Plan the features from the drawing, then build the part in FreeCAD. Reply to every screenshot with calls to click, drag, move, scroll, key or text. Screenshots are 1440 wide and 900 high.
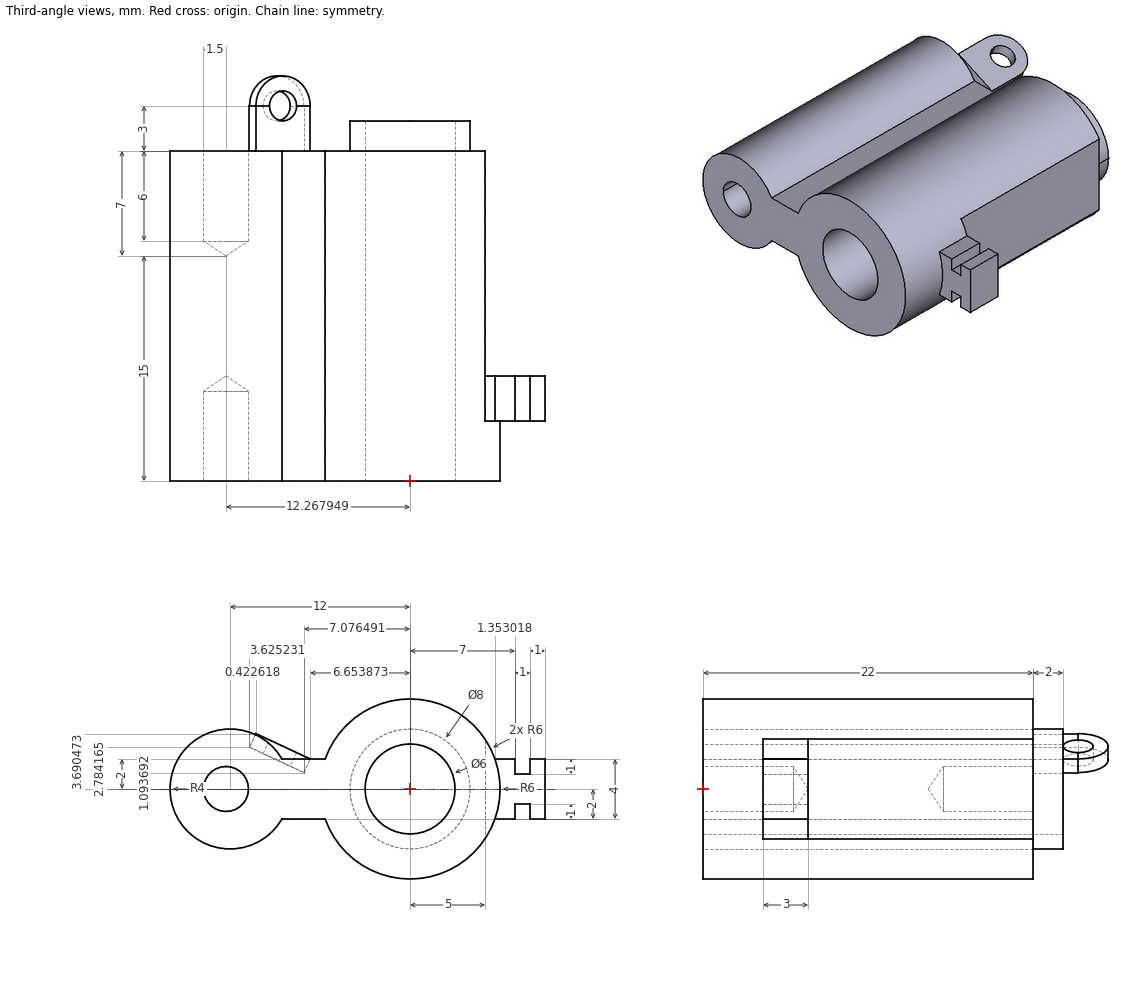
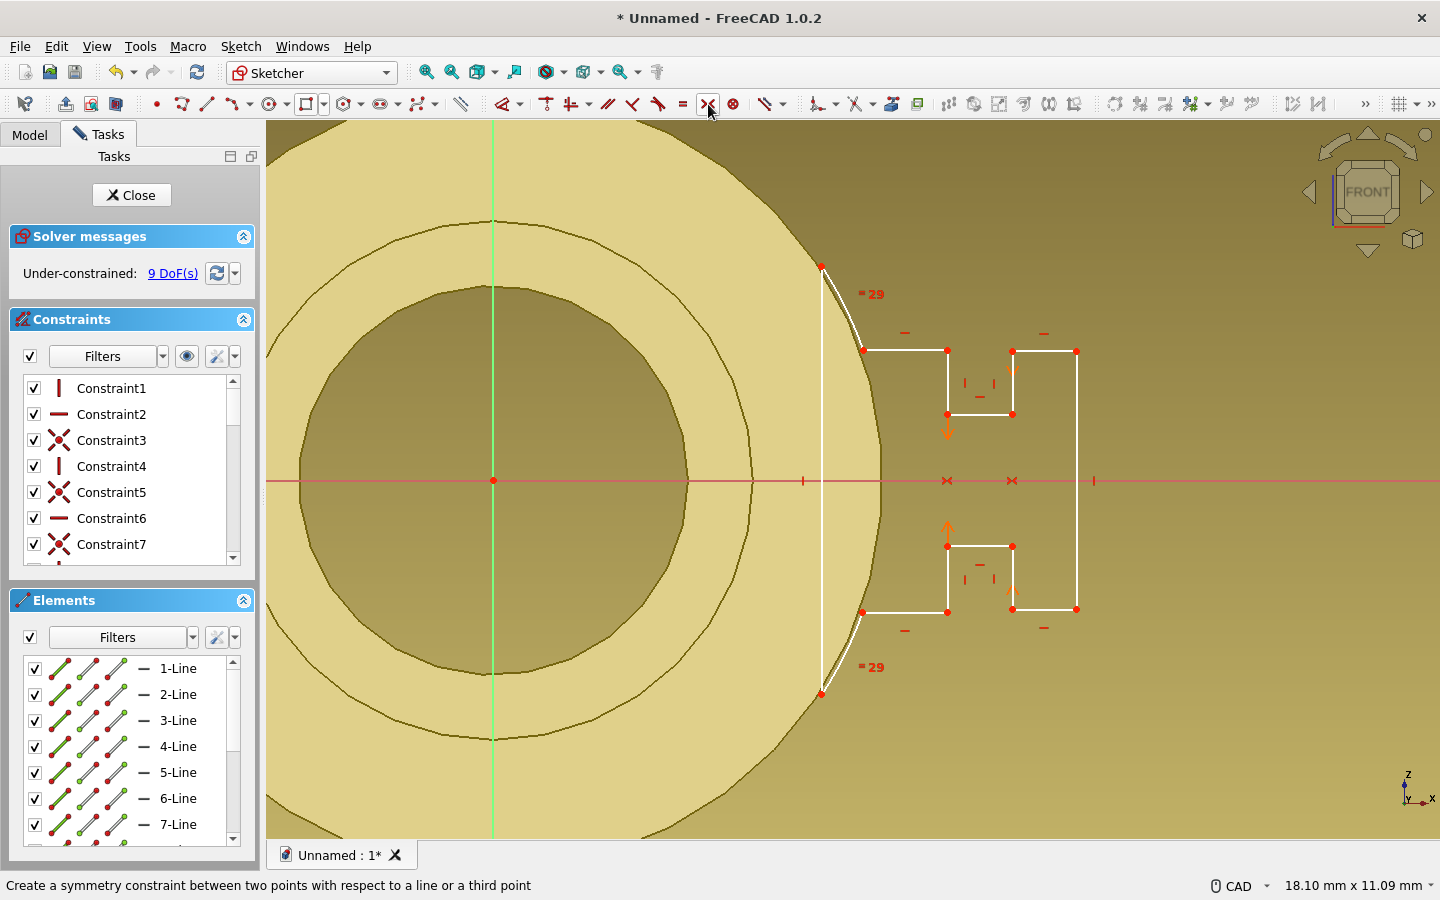
click(502, 104)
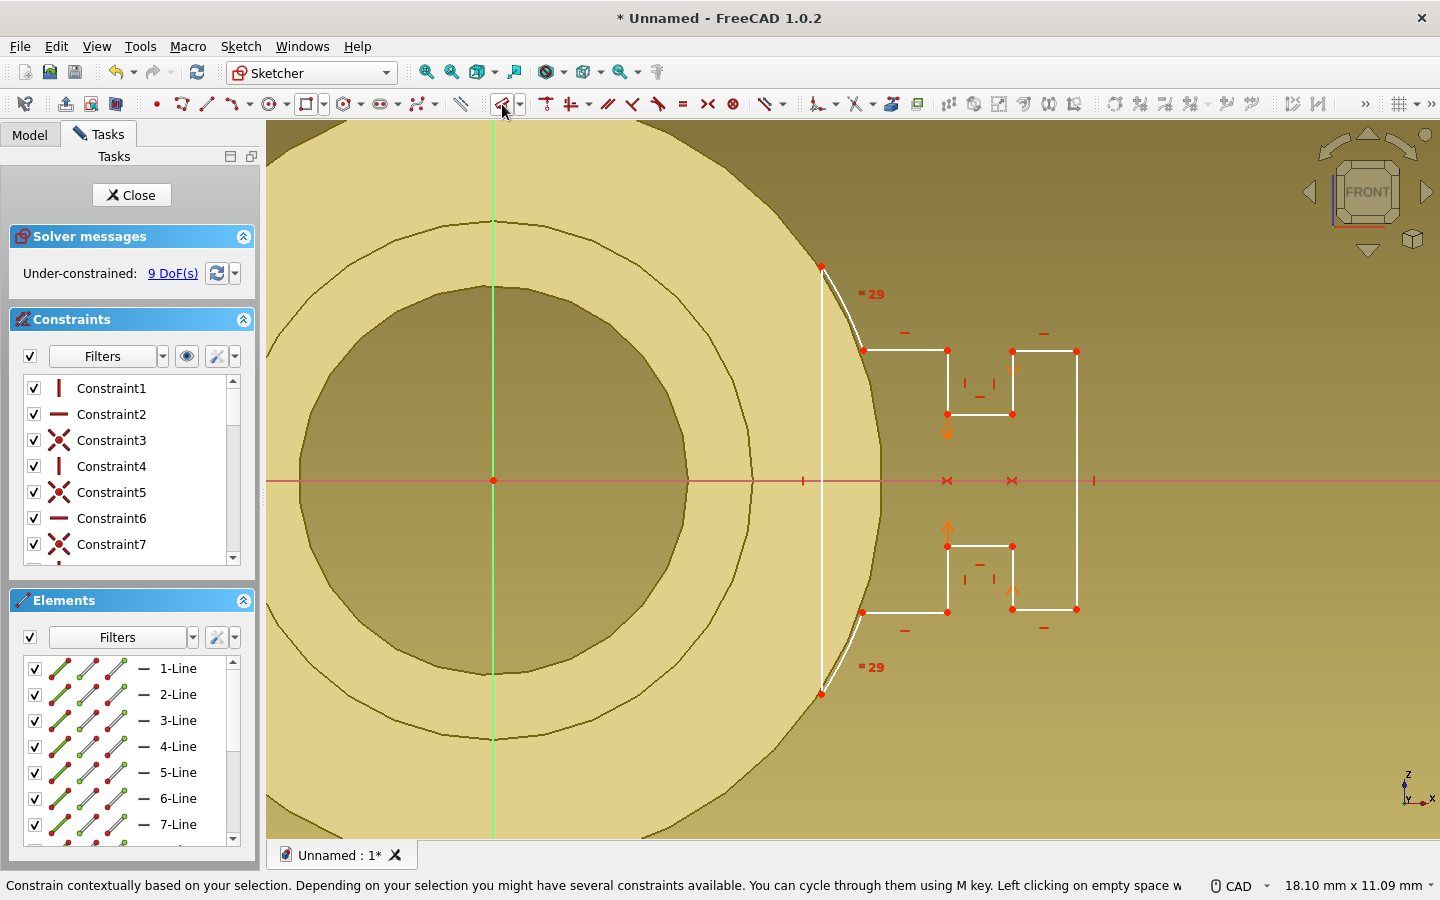
click(853, 324)
click(882, 311)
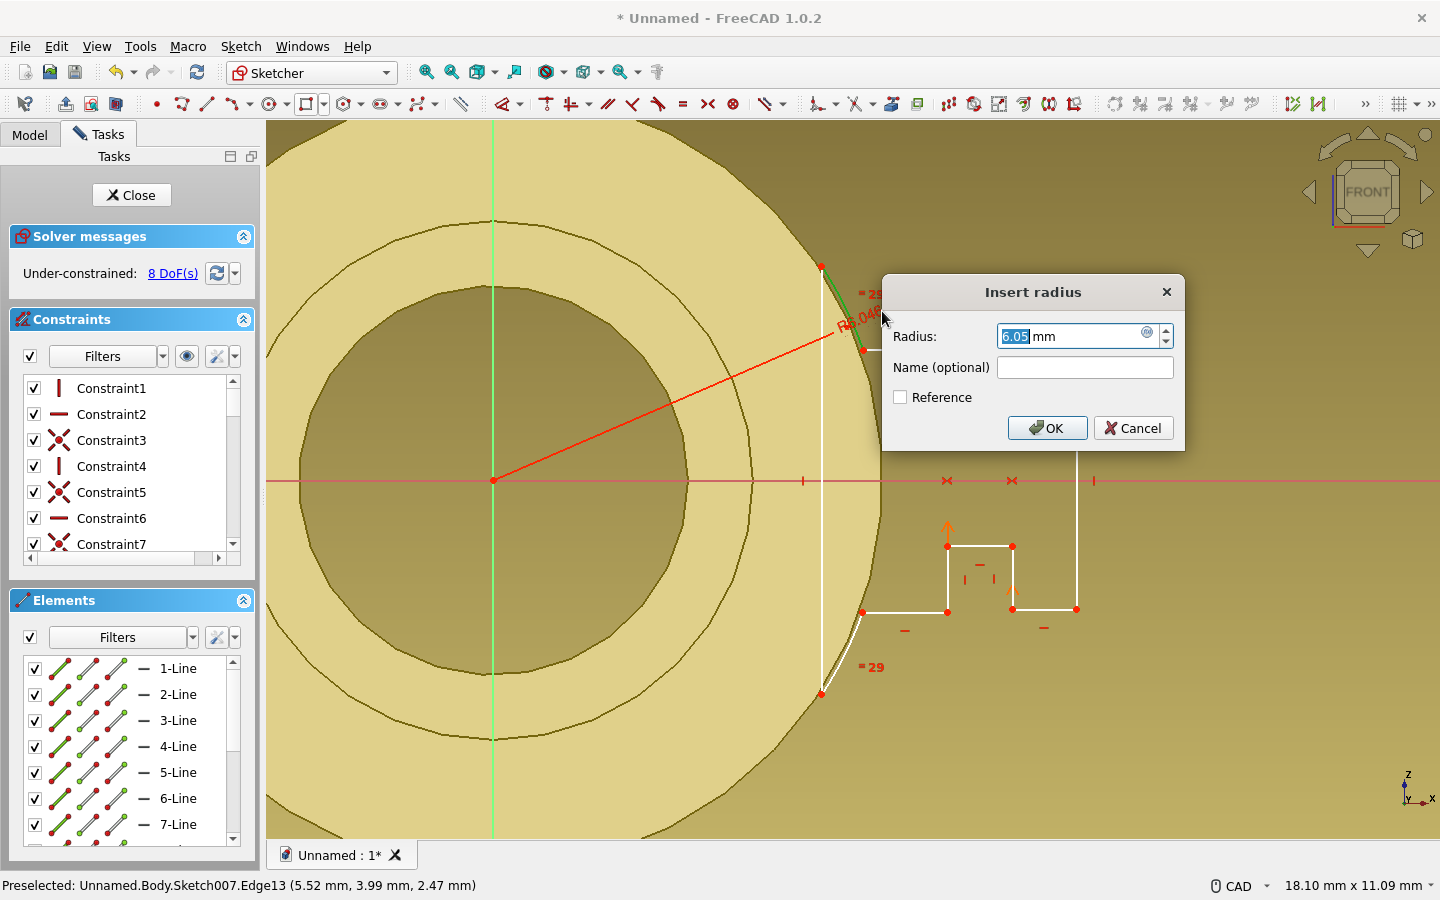
text(6)
key(Return)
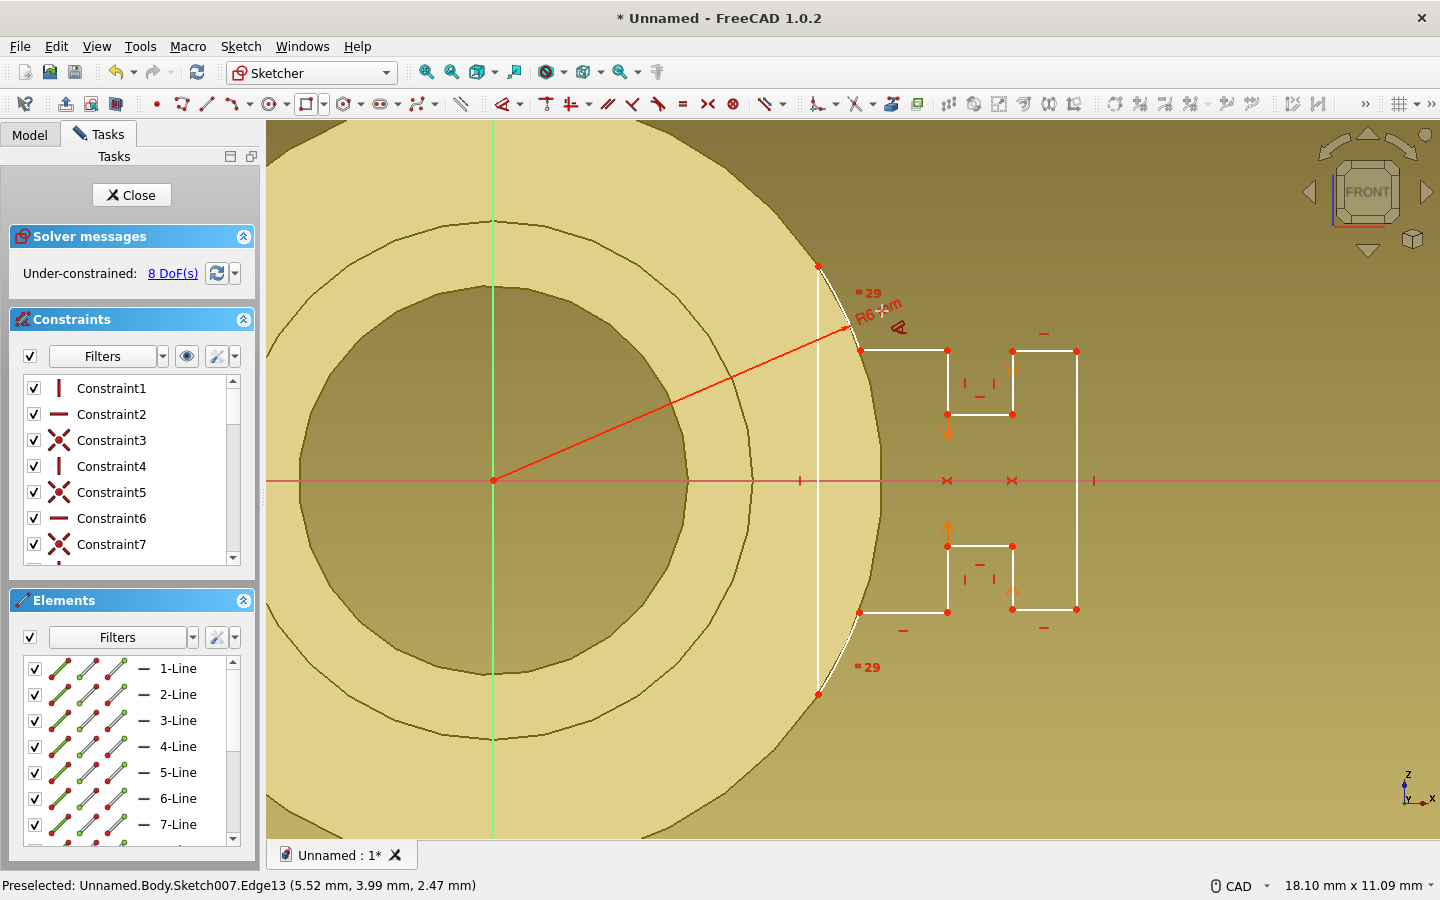
click(967, 415)
click(980, 381)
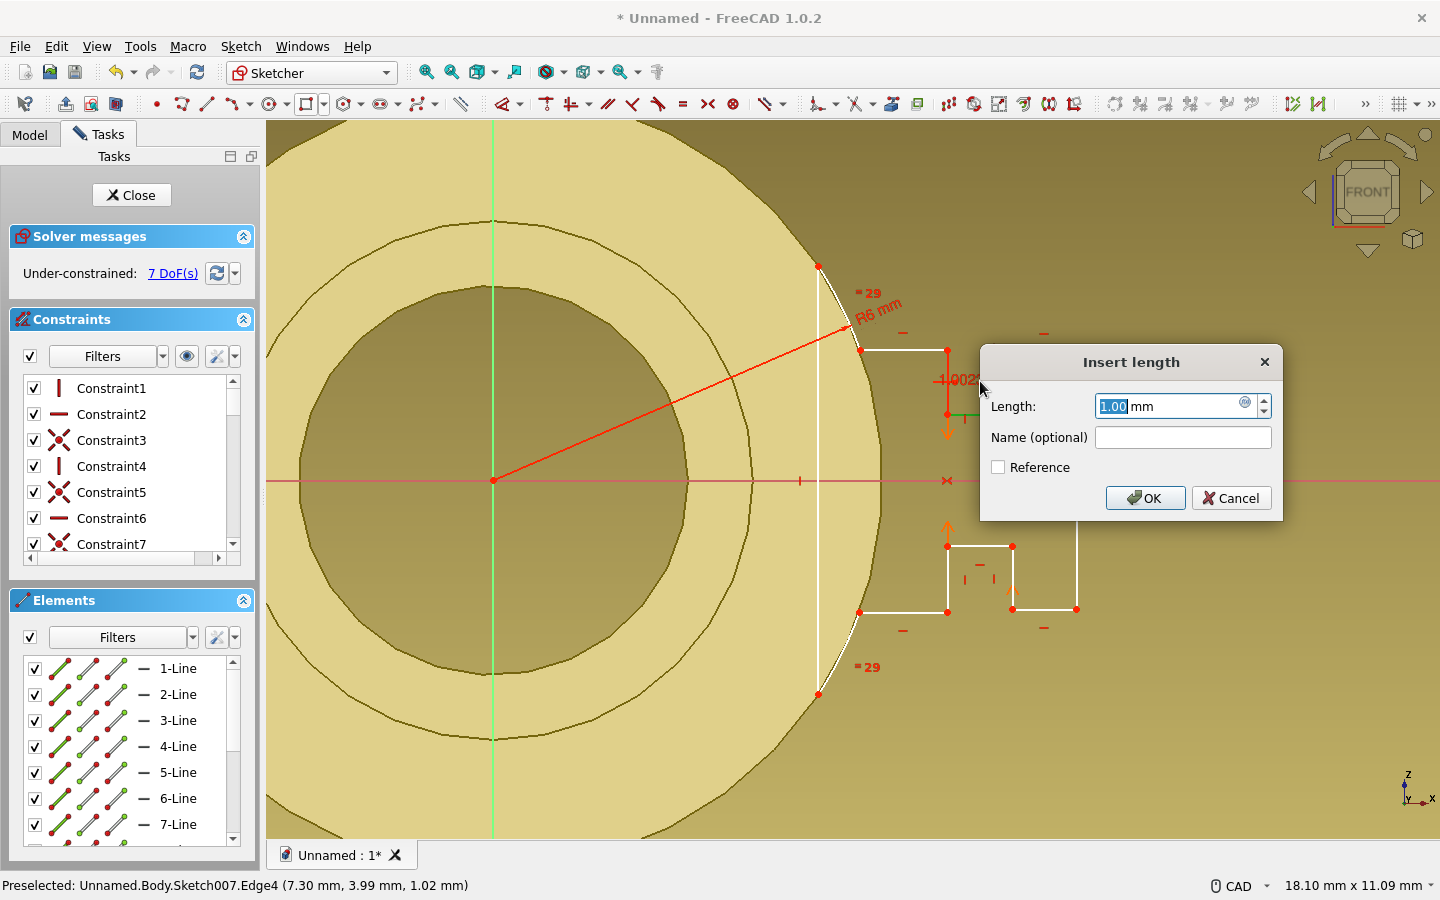
text(1)
key(Return)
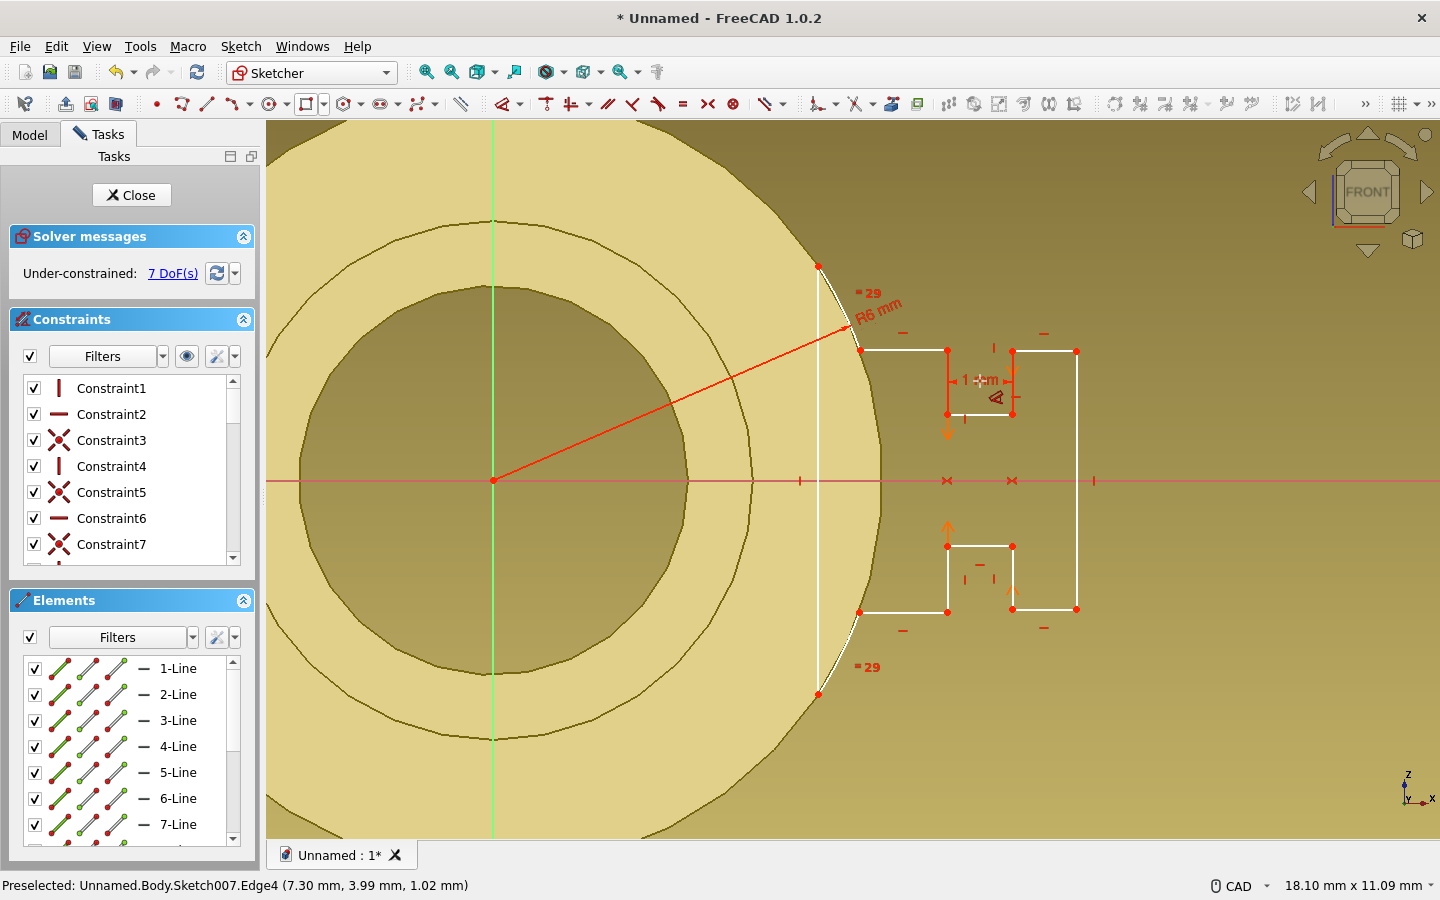
click(1013, 396)
click(1047, 405)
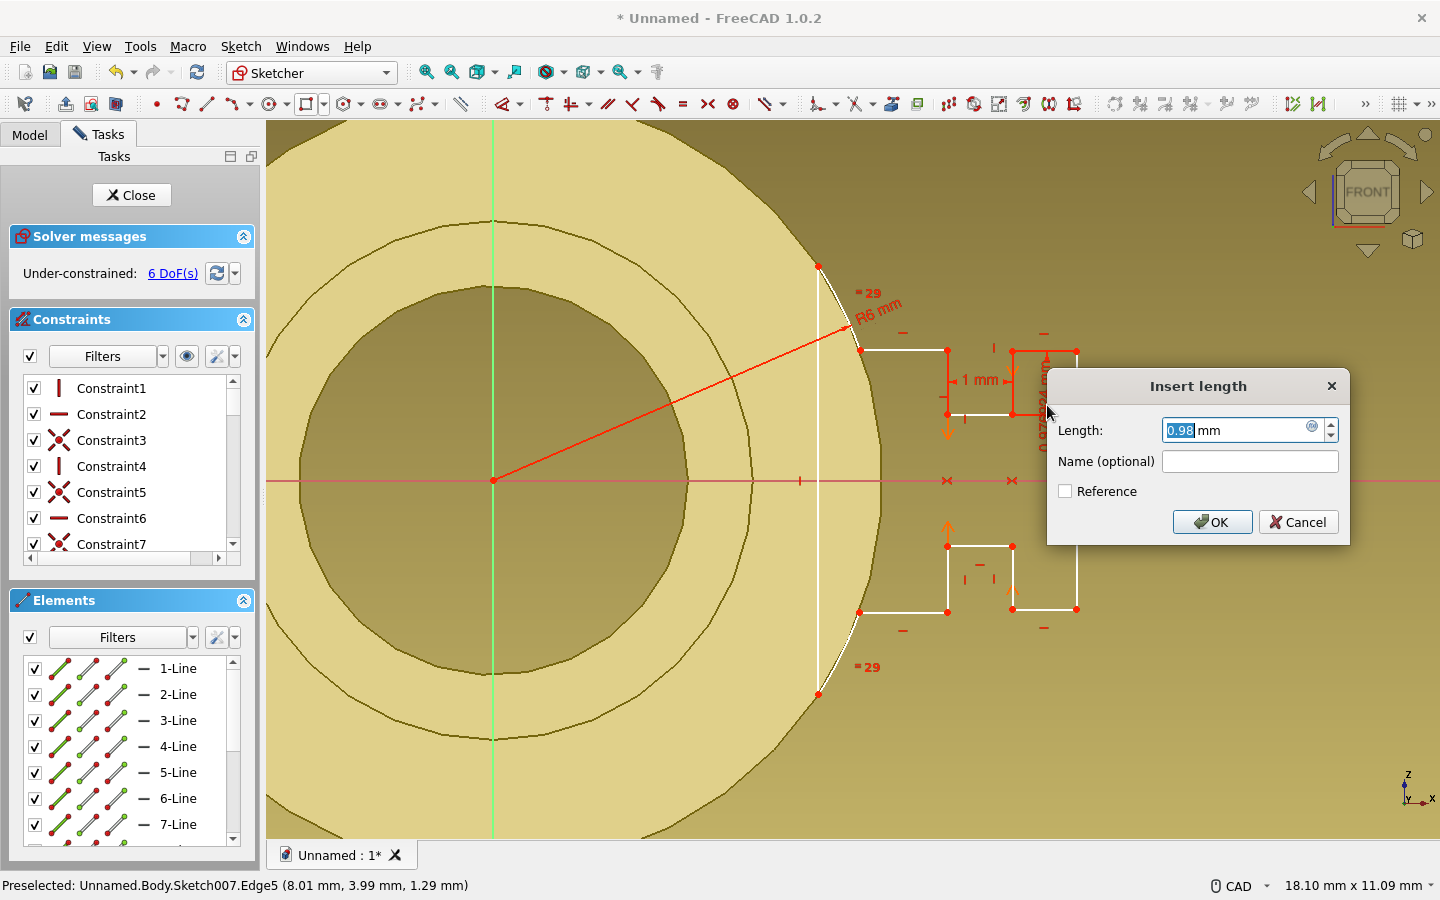
text(1)
key(Return)